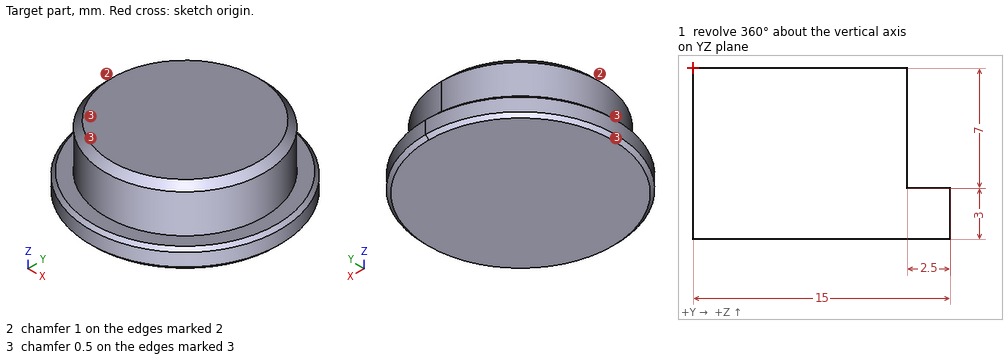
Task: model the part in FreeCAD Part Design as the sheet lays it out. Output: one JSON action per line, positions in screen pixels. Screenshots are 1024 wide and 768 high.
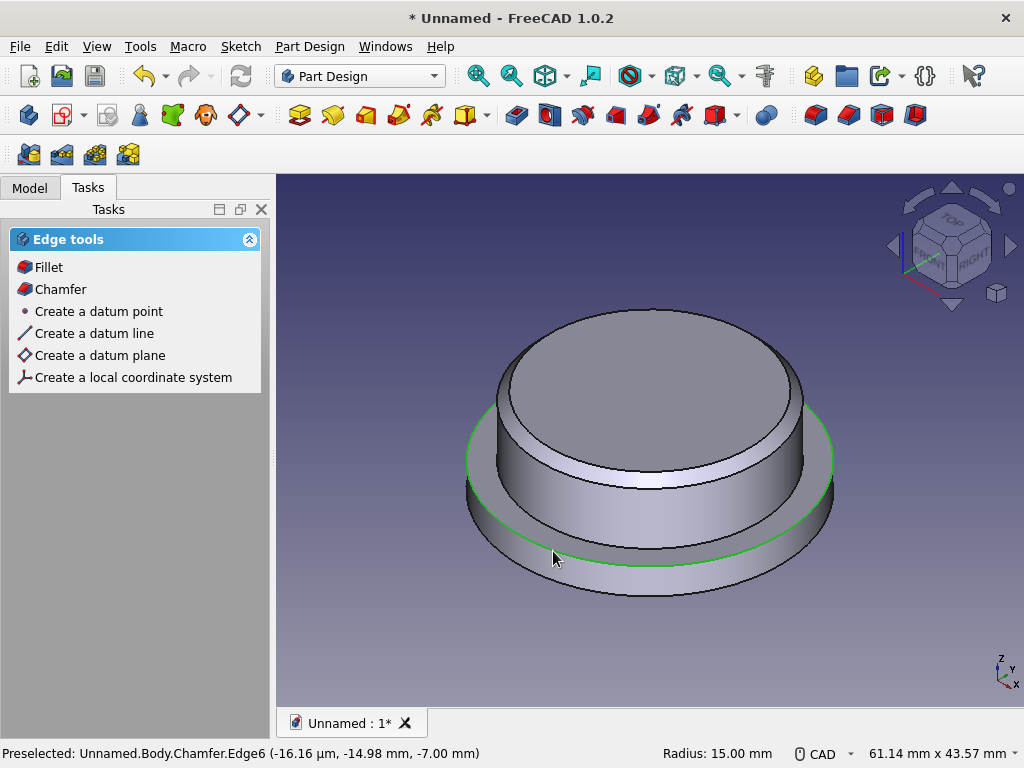
{"action": "key", "text": "2"}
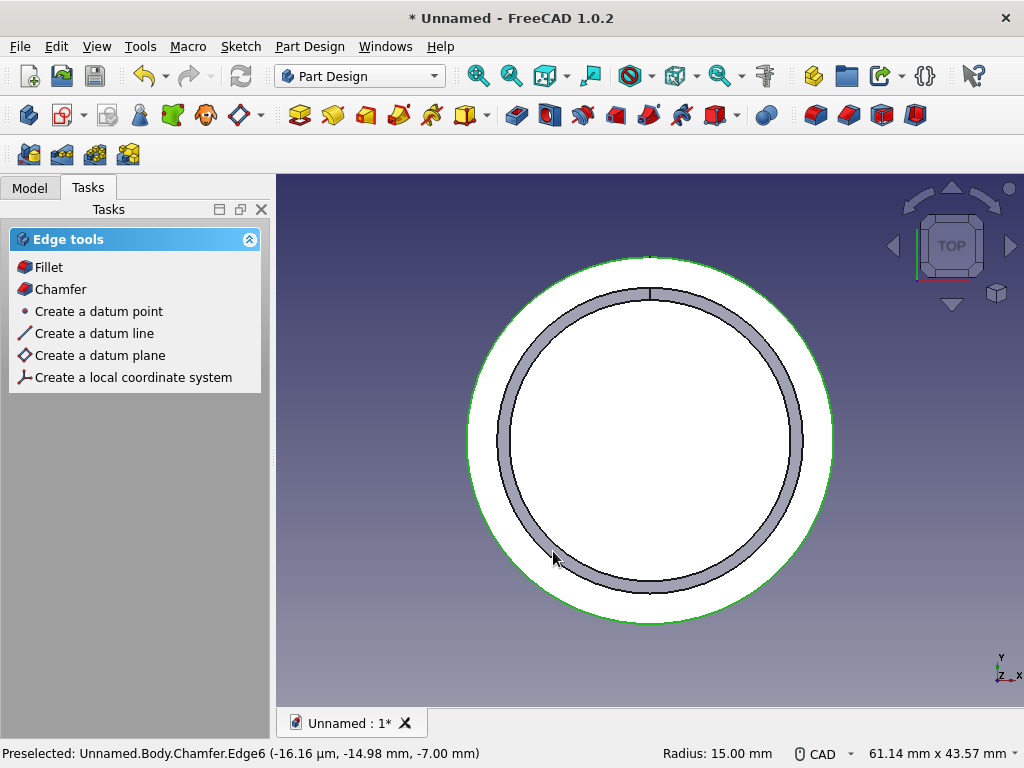
{"action": "key", "text": "1"}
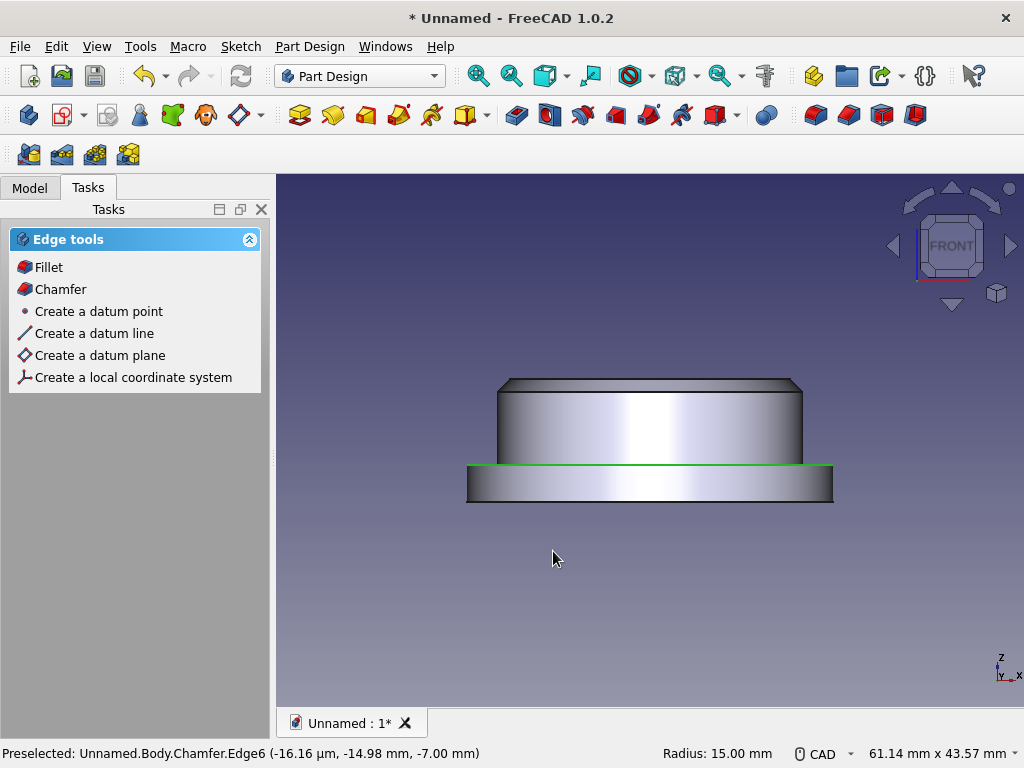
{"action": "left_click", "coordinate": [650, 501], "text": "ctrl"}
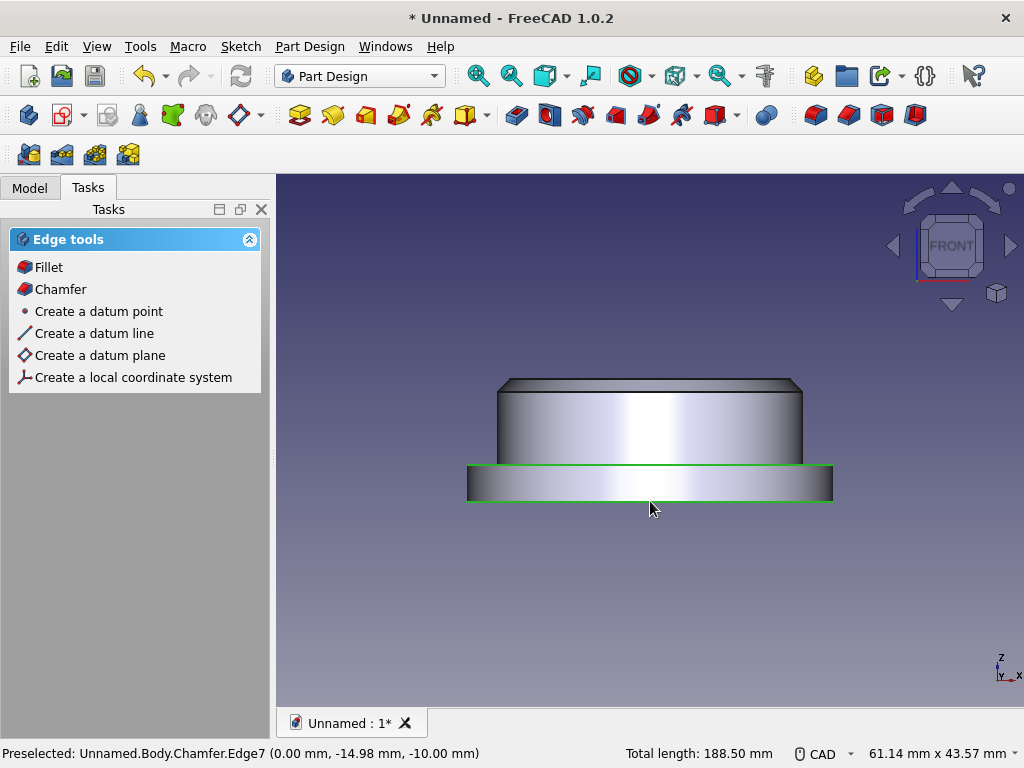
{"action": "left_click", "coordinate": [849, 116]}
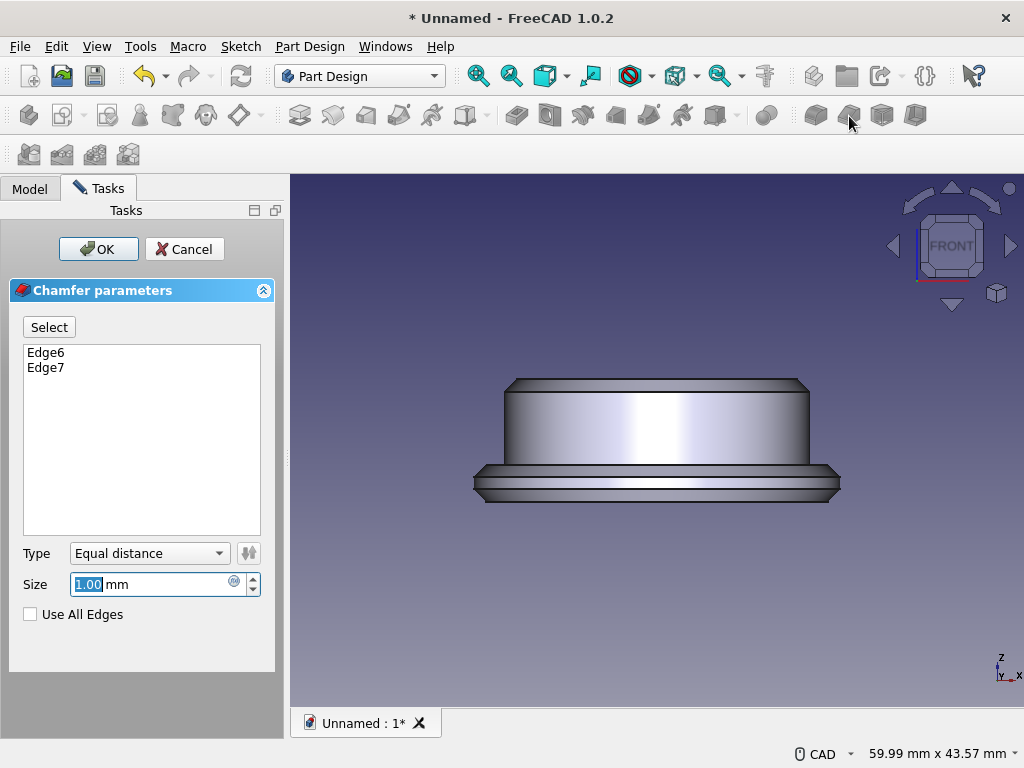
{"action": "type", "text": "0.5"}
{"action": "key", "text": "Tab"}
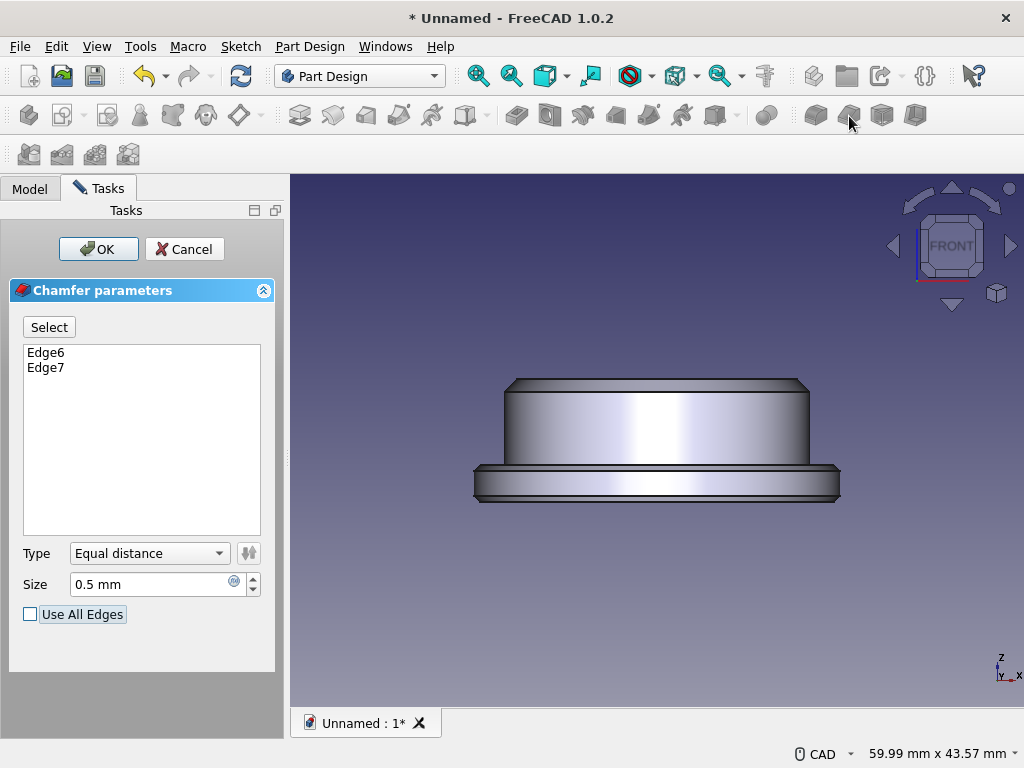
{"action": "left_click", "coordinate": [99, 249]}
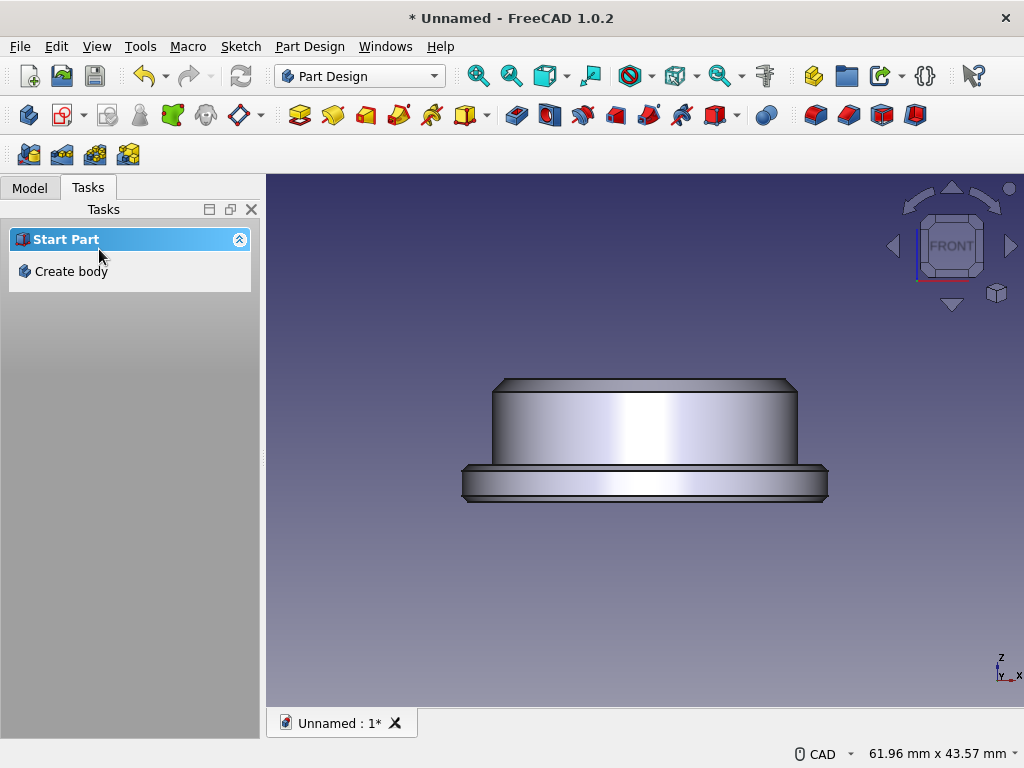
{"action": "key", "text": "0"}